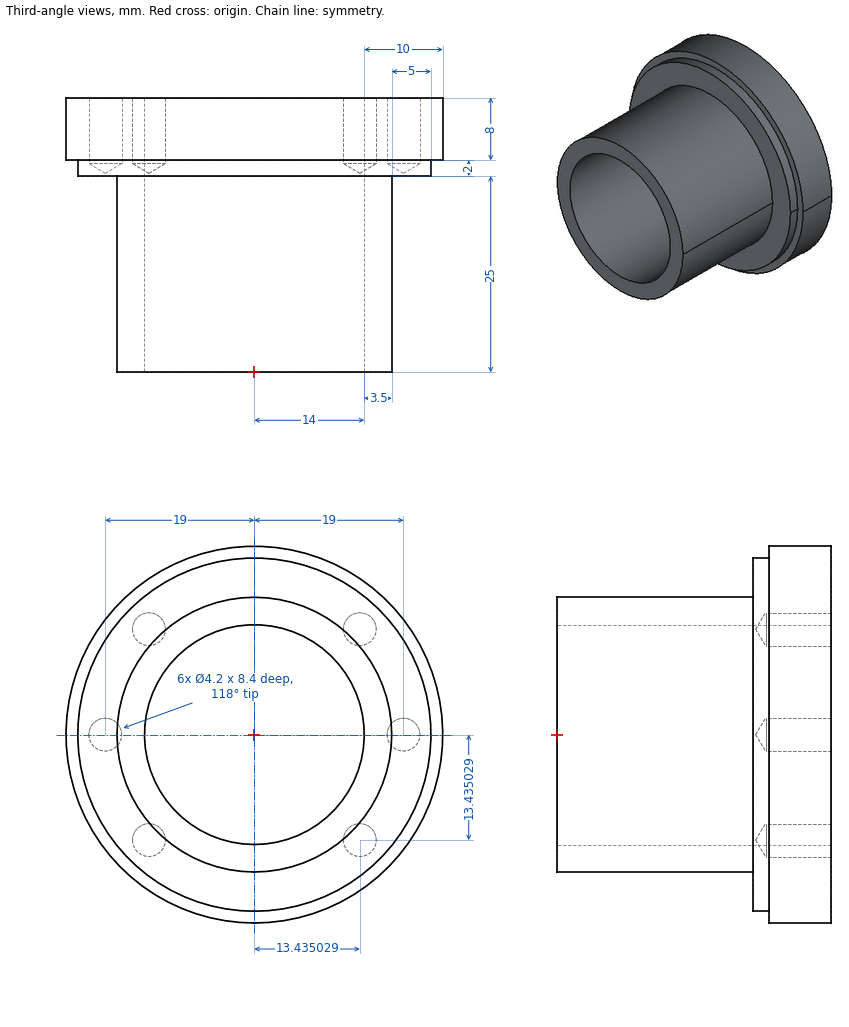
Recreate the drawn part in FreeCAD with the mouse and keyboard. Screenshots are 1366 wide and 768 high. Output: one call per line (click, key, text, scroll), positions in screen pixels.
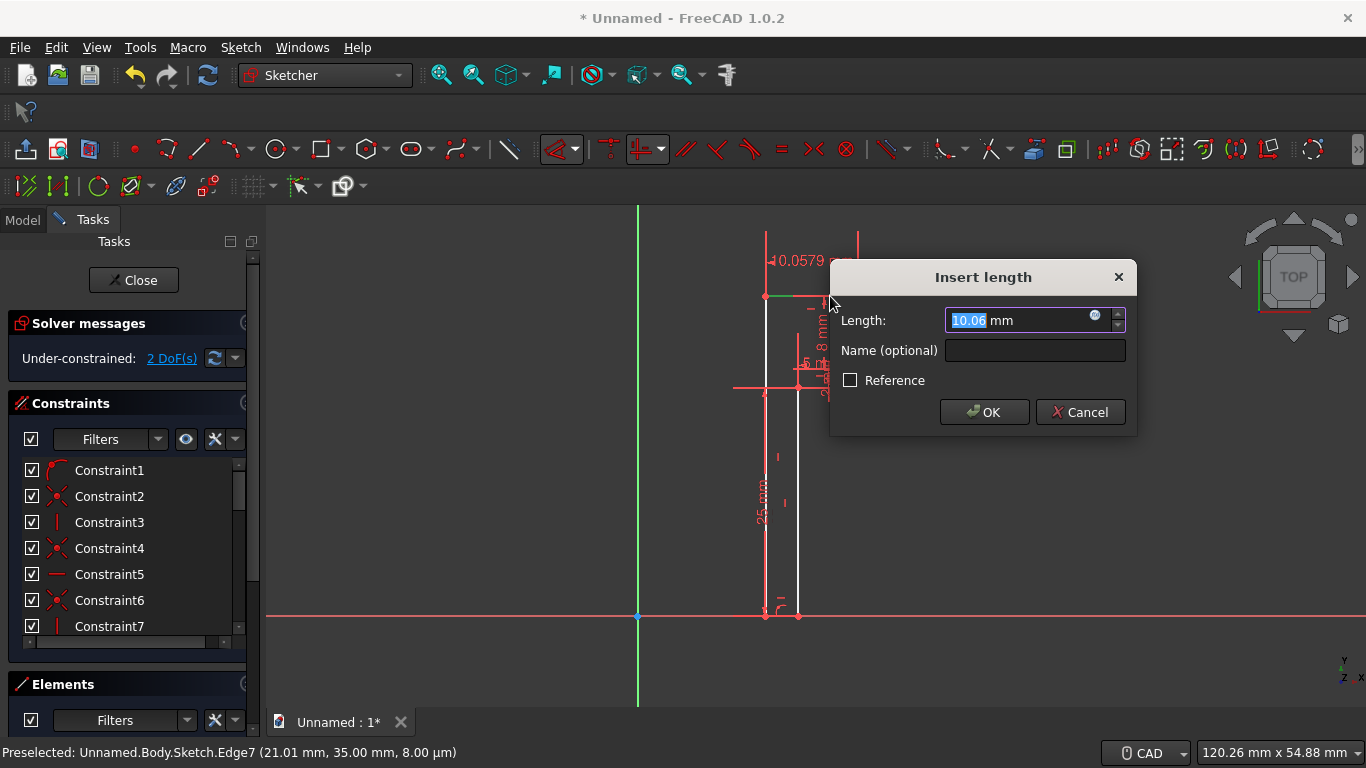
text(10)
key(Return)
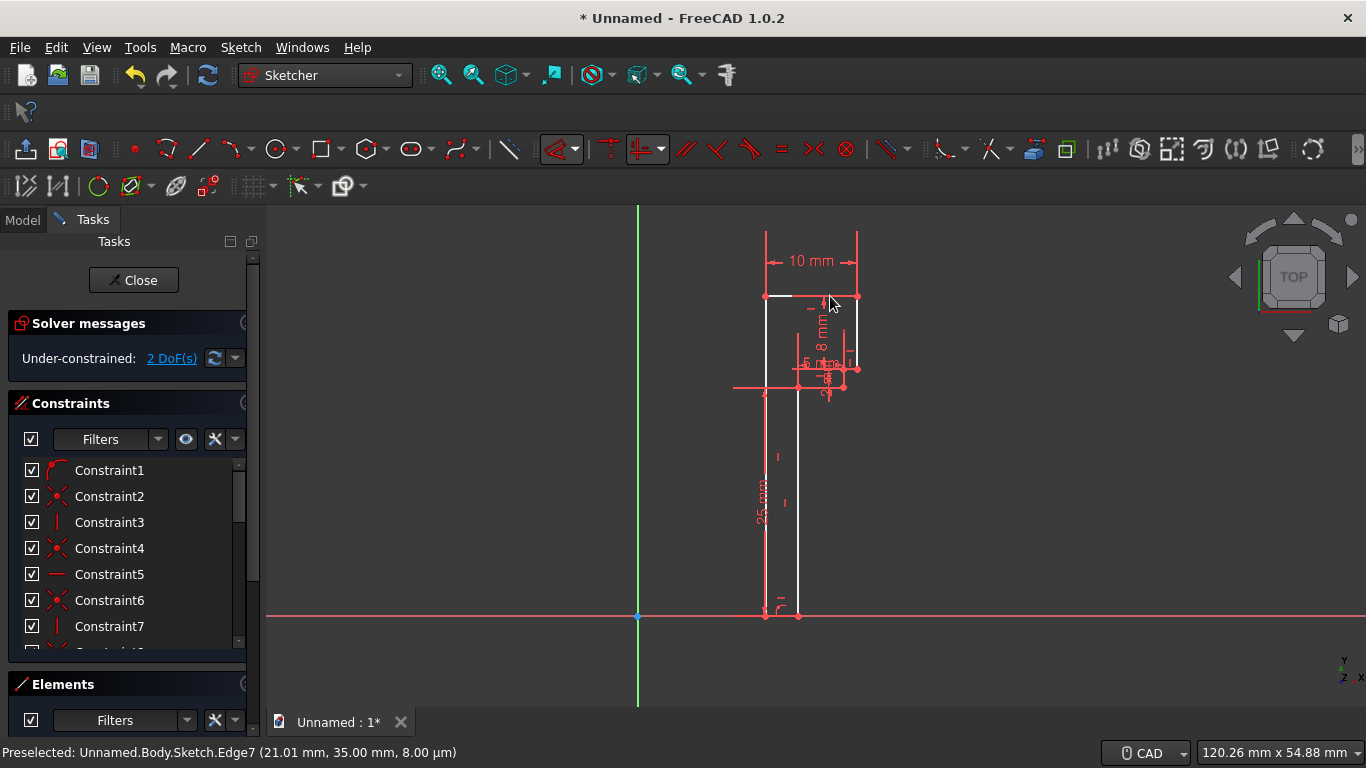
scroll(775, 616, up, 2)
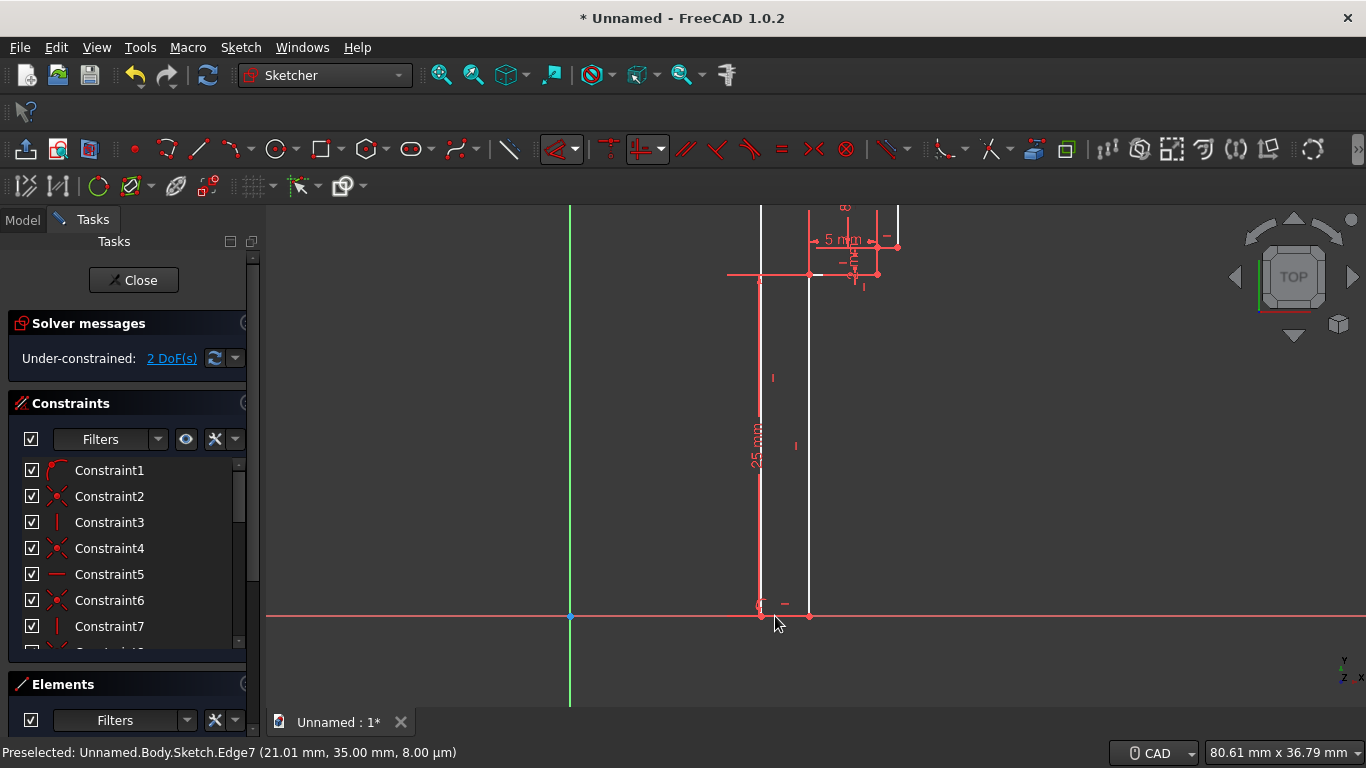
click(776, 616)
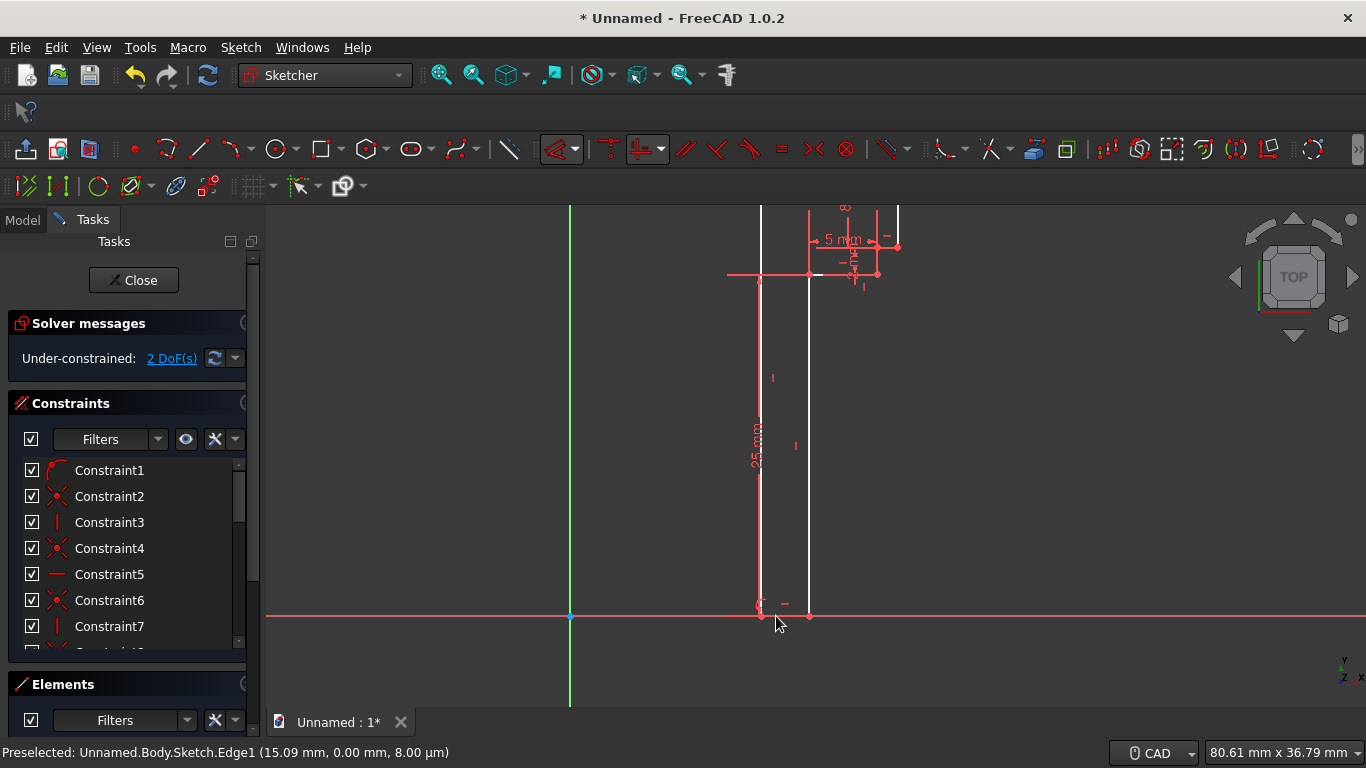
click(578, 150)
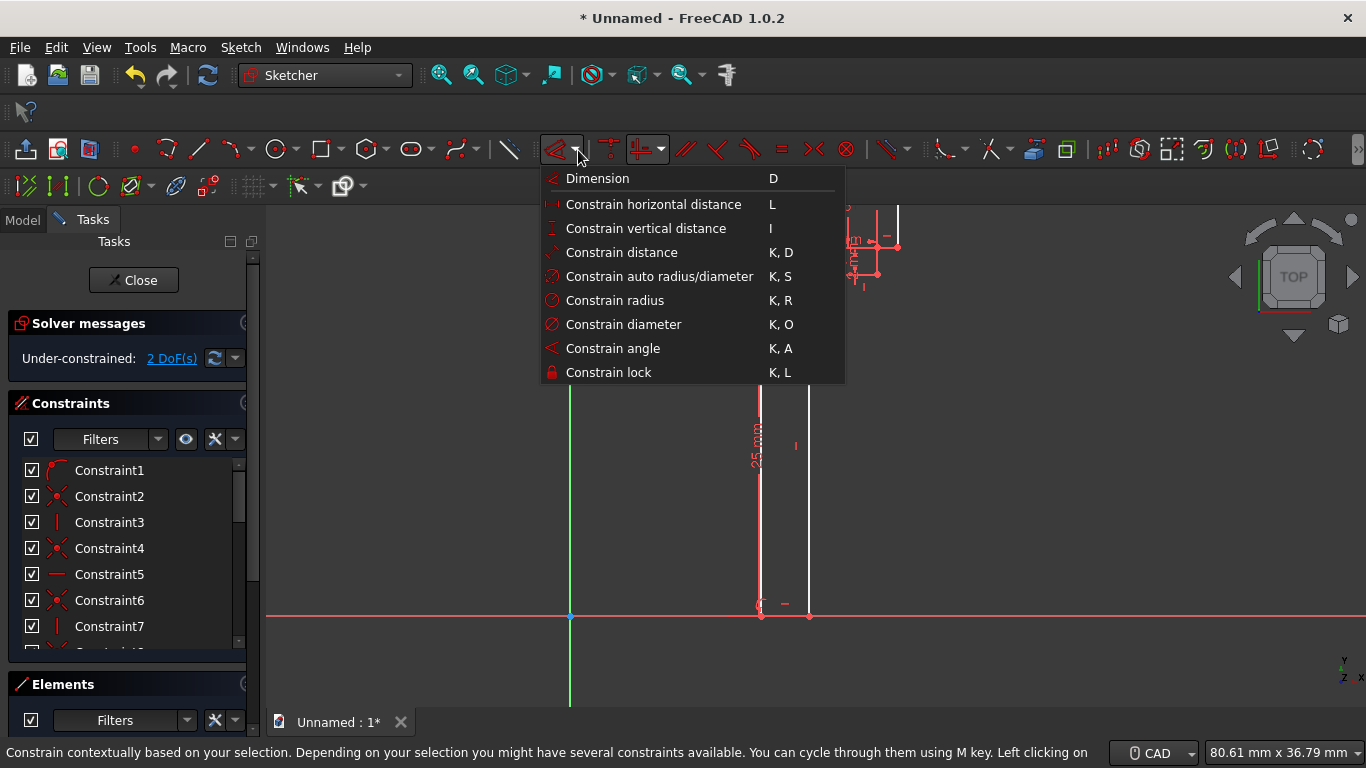
click(693, 204)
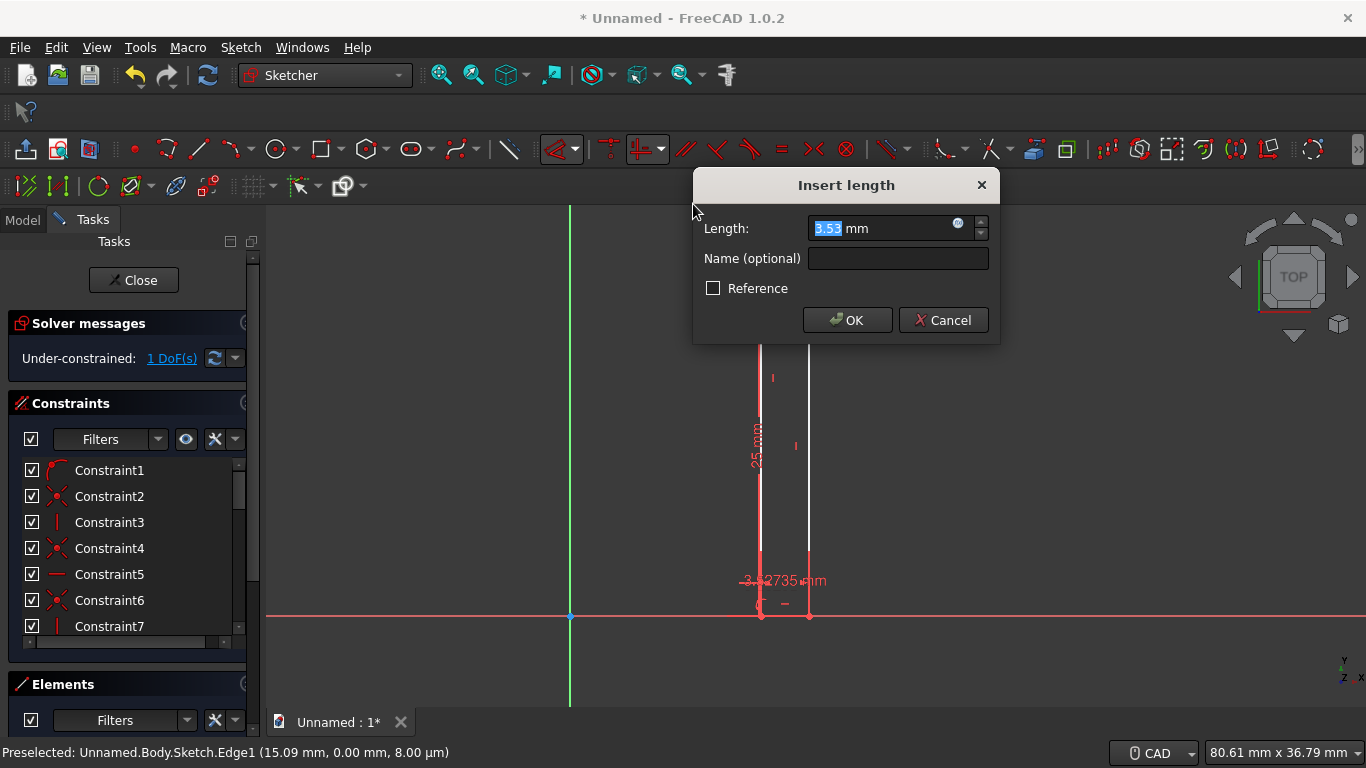
text(3.5)
key(Return)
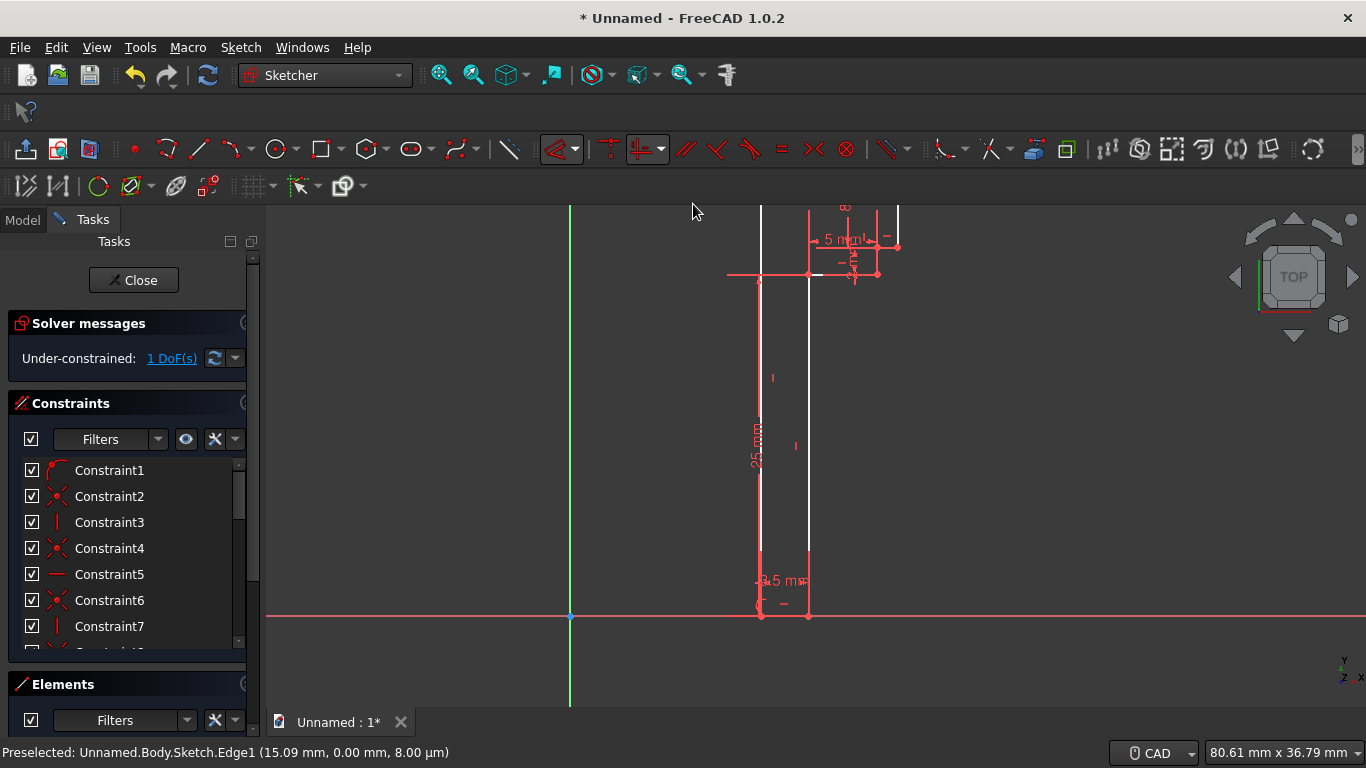
click(761, 616)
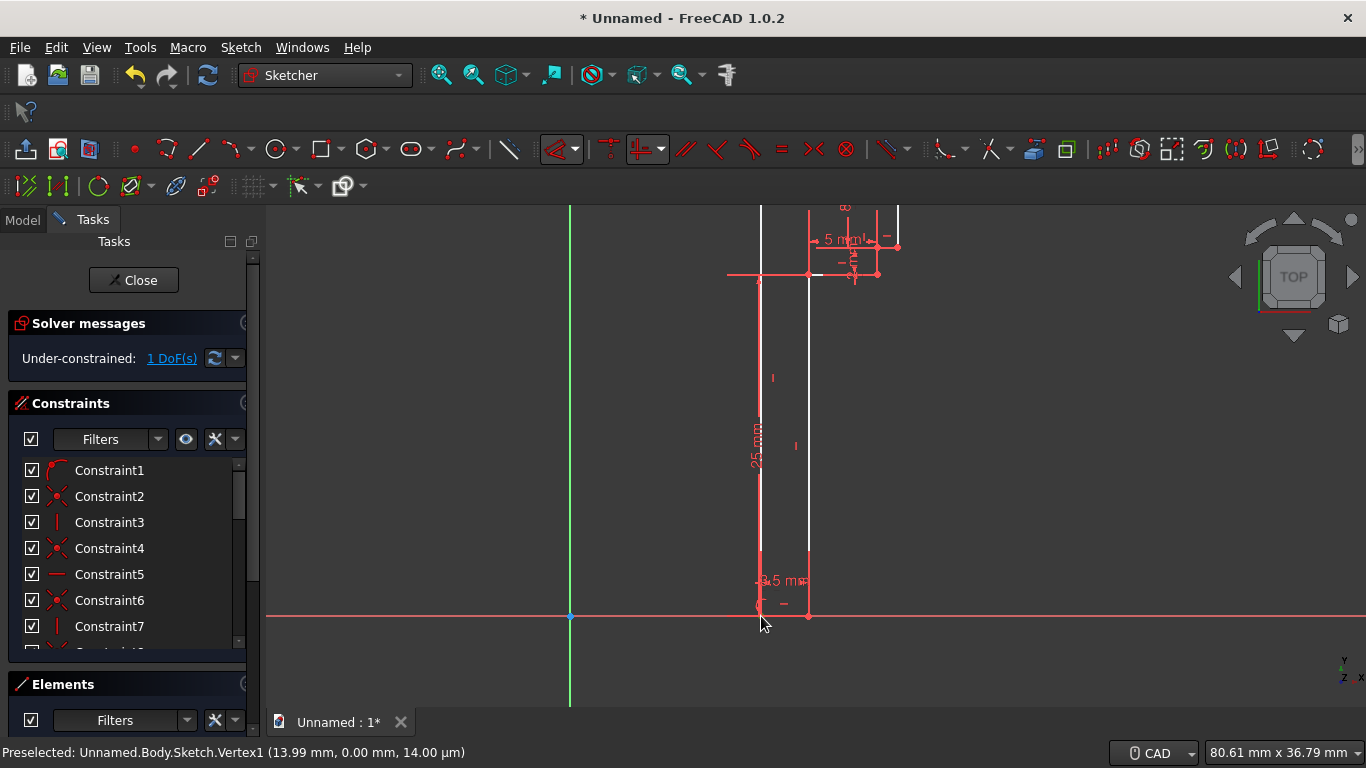
click(578, 150)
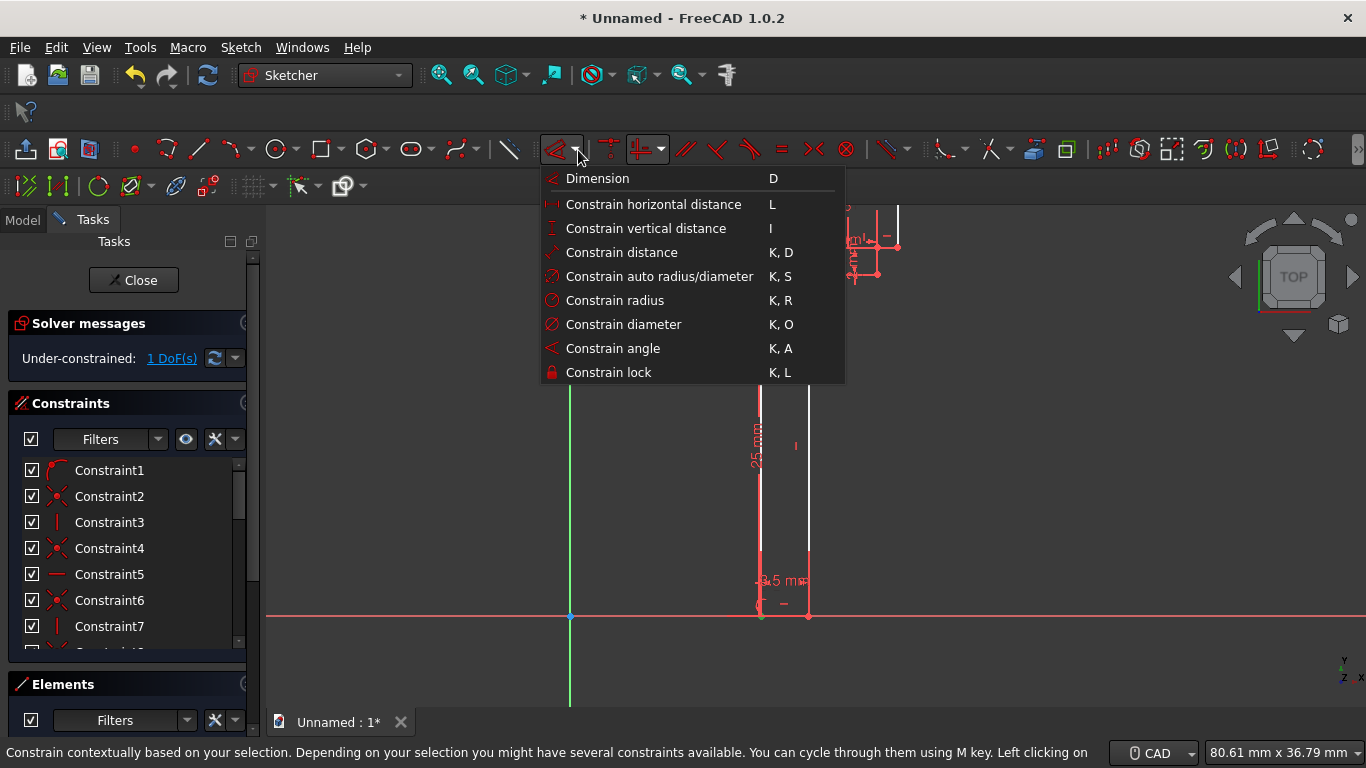
click(693, 204)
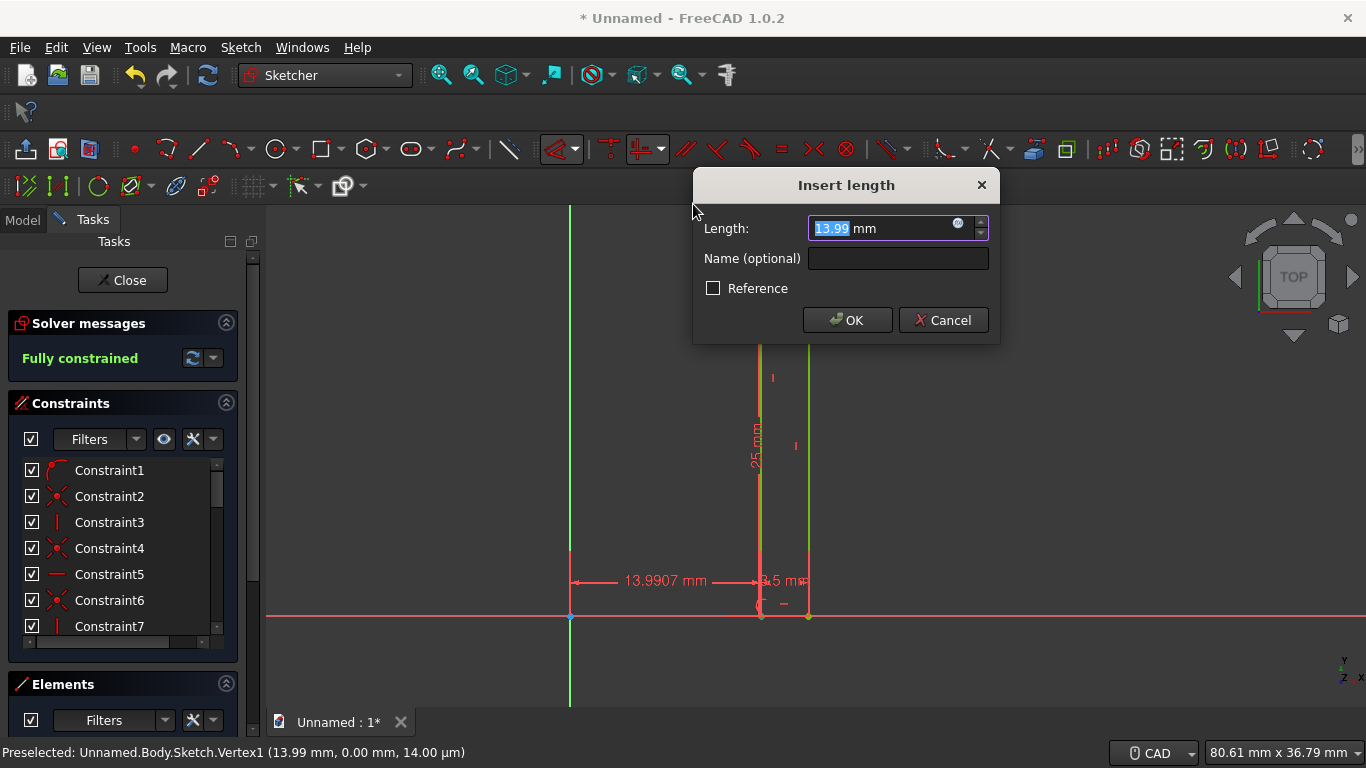
text(14)
key(Return)